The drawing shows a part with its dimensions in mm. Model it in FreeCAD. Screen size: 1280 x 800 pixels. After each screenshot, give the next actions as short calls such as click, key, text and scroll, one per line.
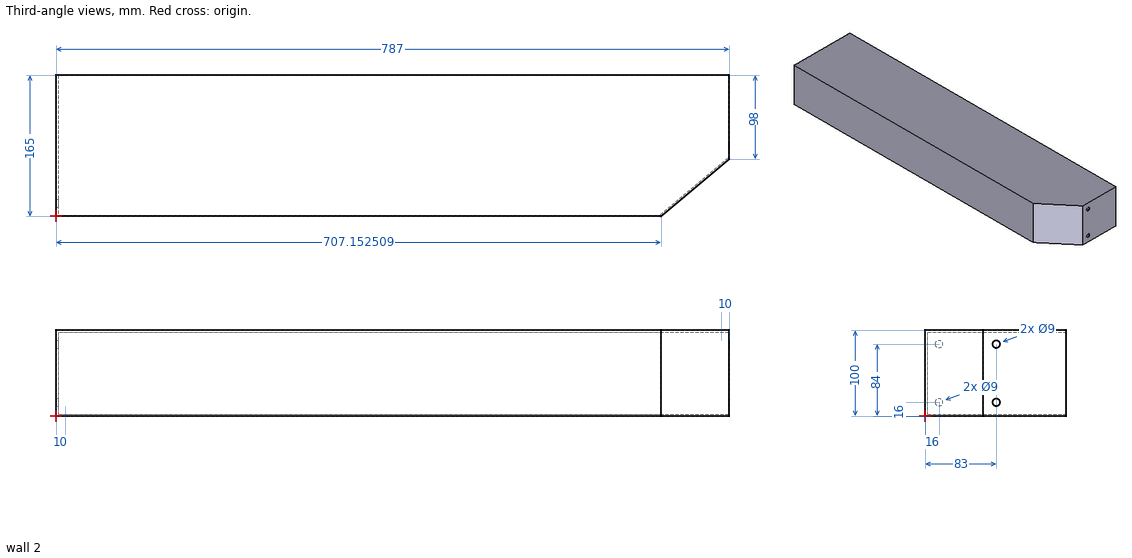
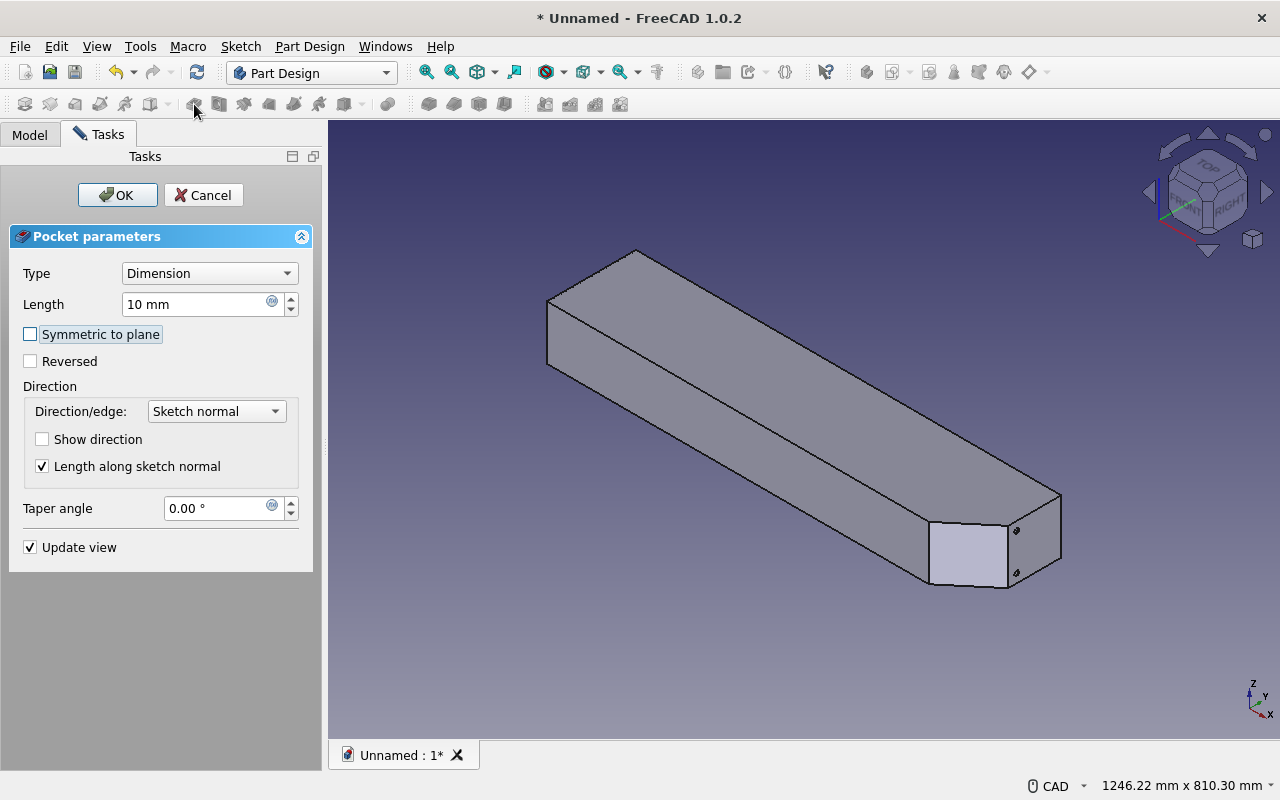
click(118, 195)